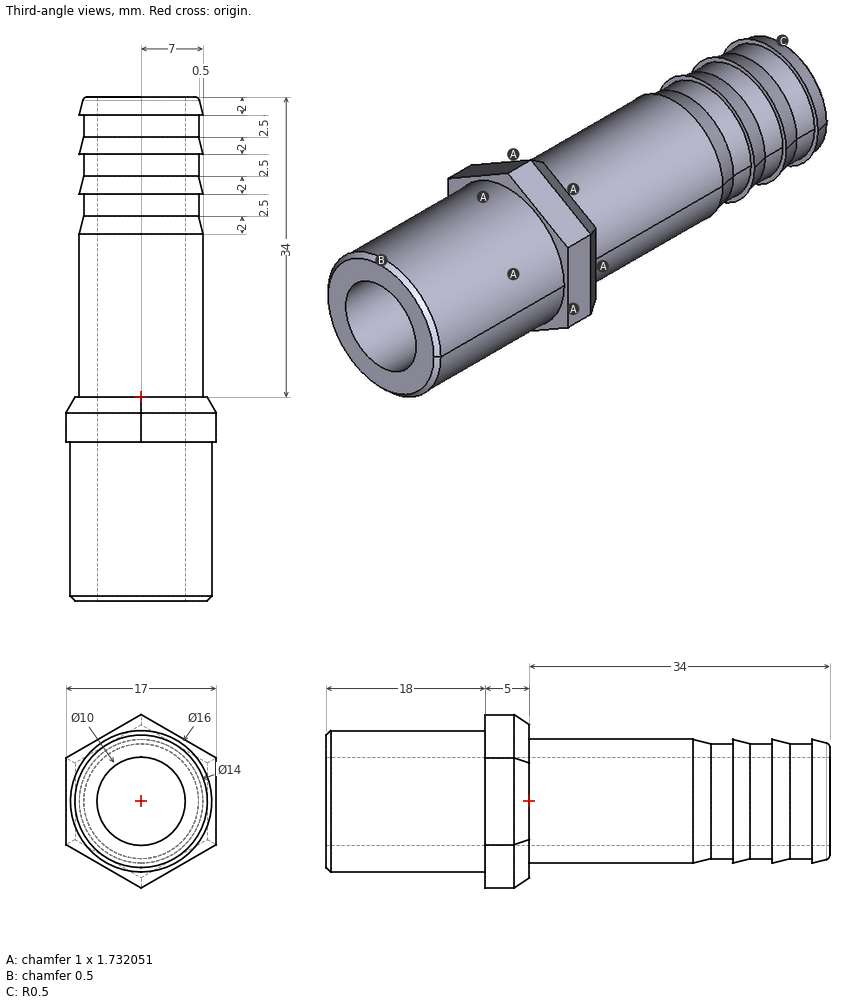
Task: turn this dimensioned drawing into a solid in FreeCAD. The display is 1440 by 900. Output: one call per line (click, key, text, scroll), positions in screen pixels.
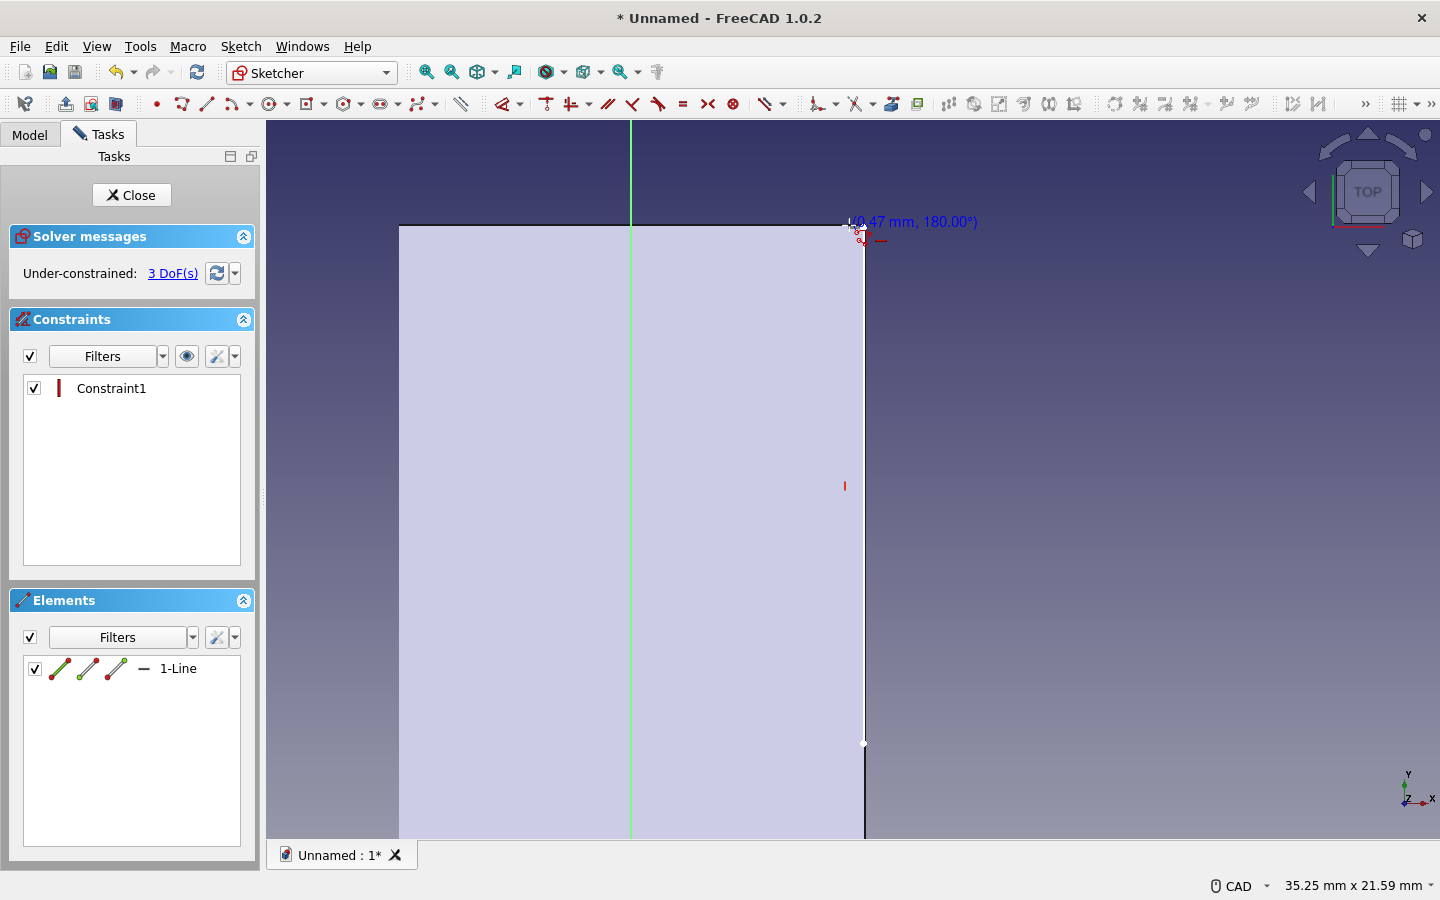
click(848, 225)
click(865, 292)
click(848, 292)
click(848, 375)
click(865, 441)
click(848, 441)
click(848, 525)
click(865, 591)
click(848, 591)
click(848, 675)
click(864, 743)
key(Escape)
key(Escape)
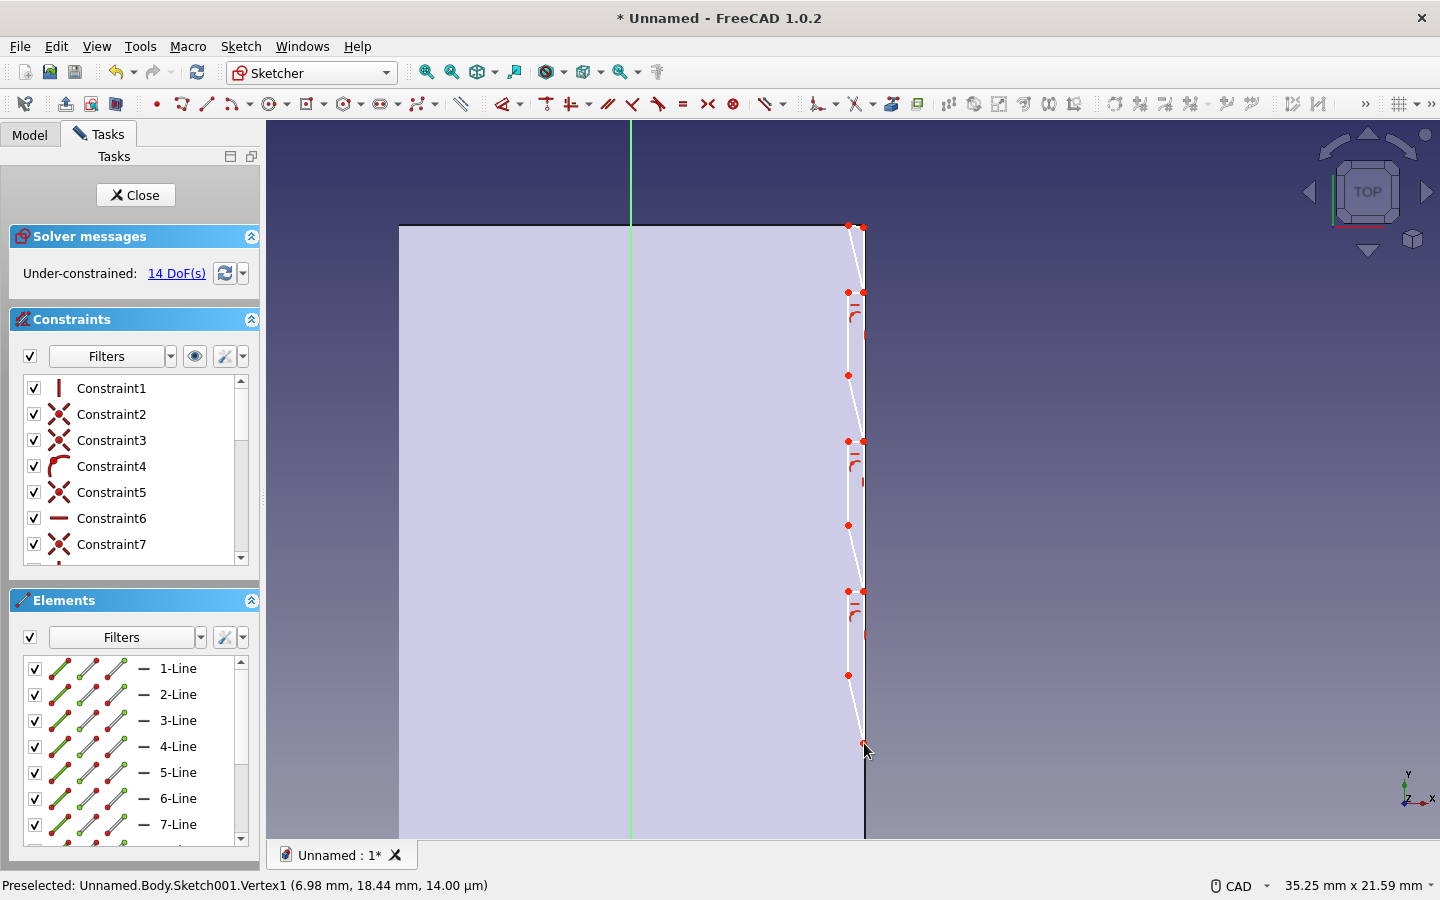
scroll(856, 227, up, 3)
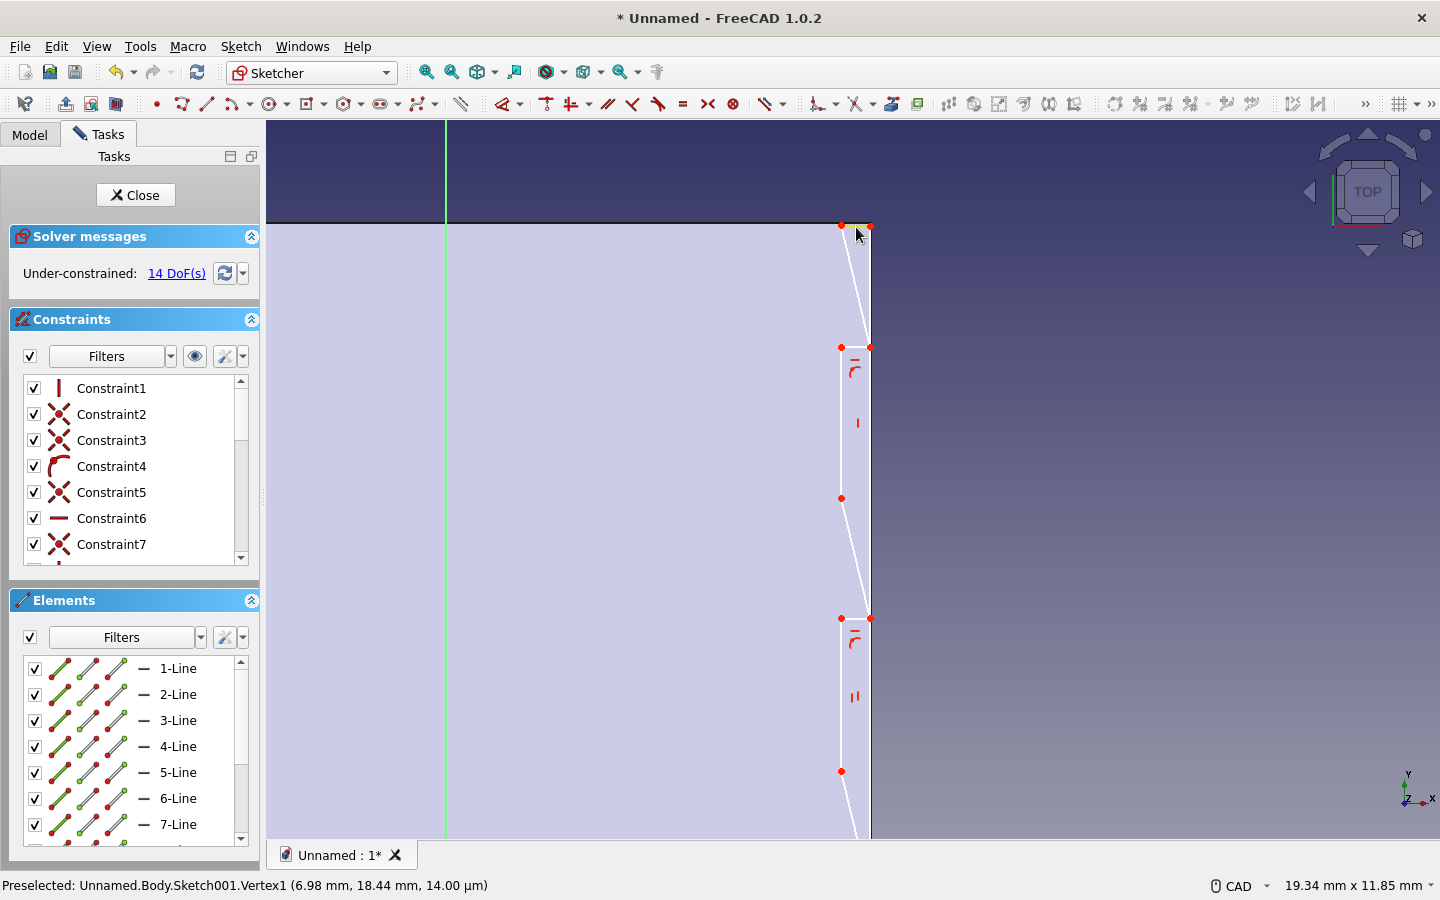
click(856, 226)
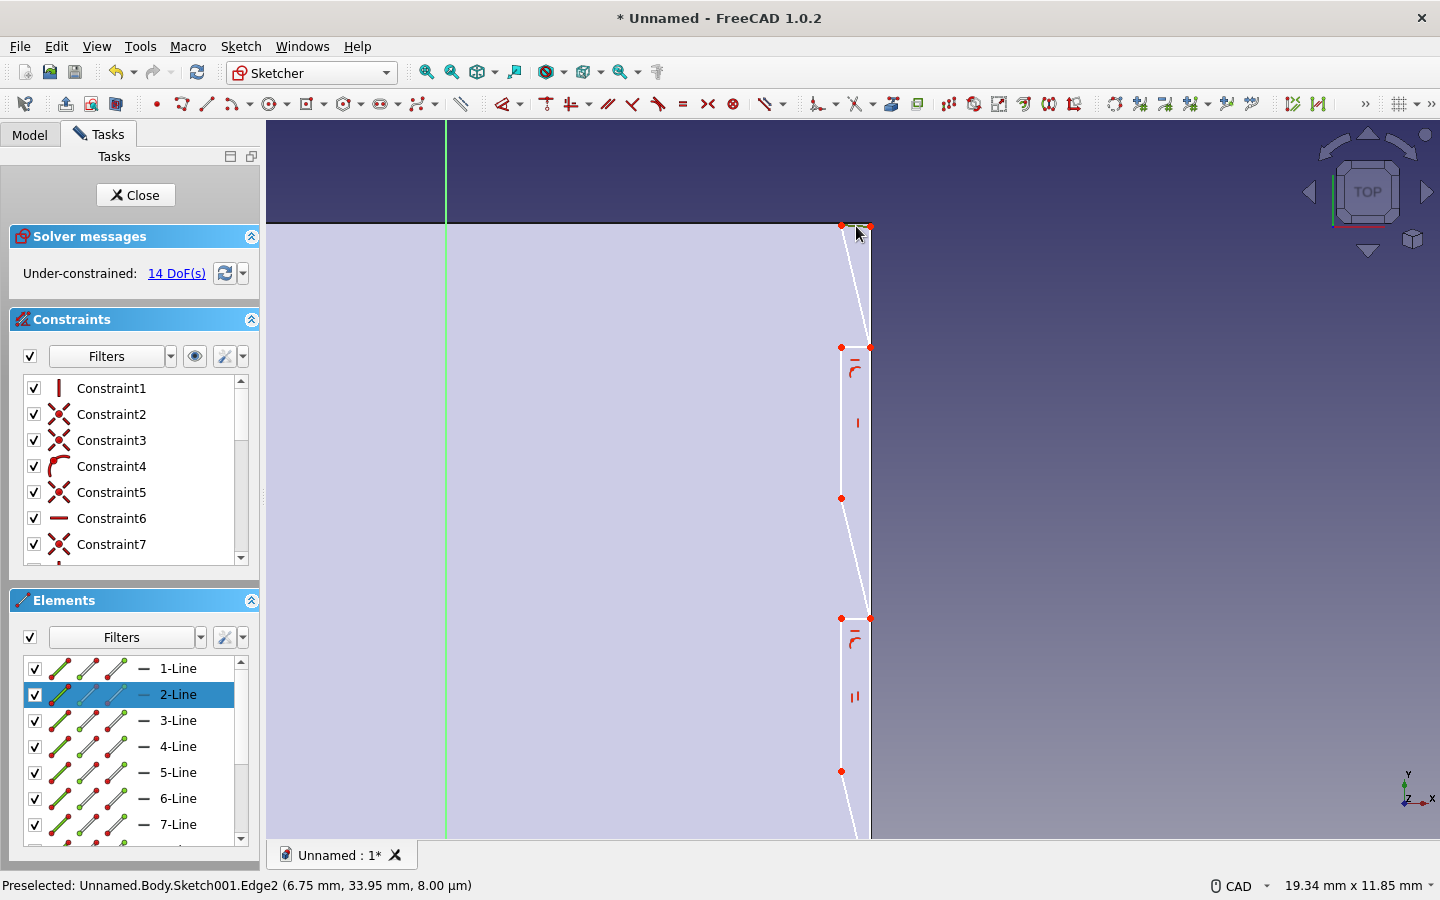
click(588, 104)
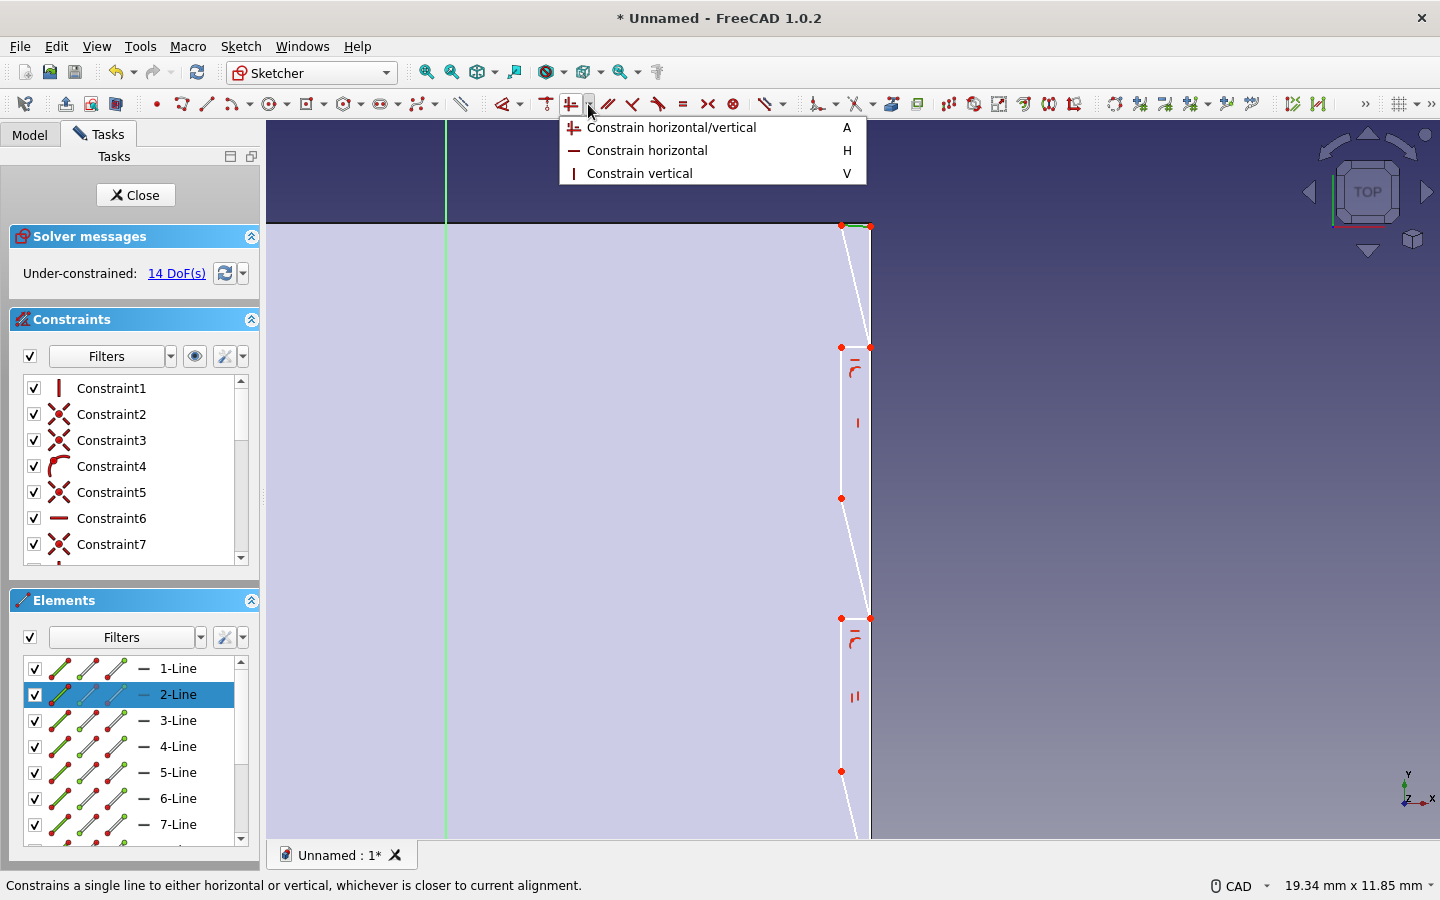
click(713, 150)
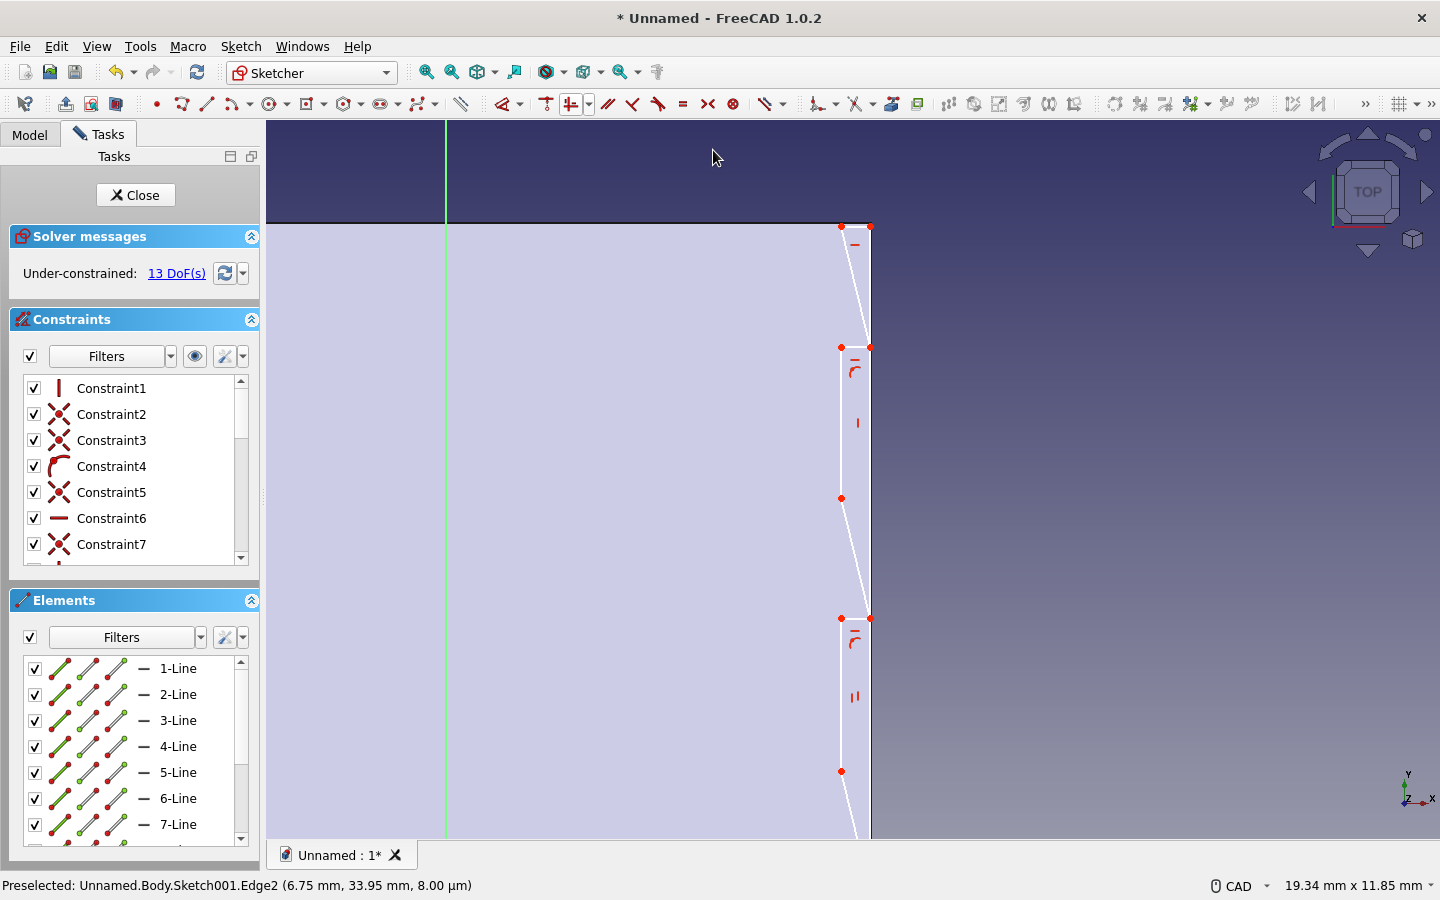
click(502, 104)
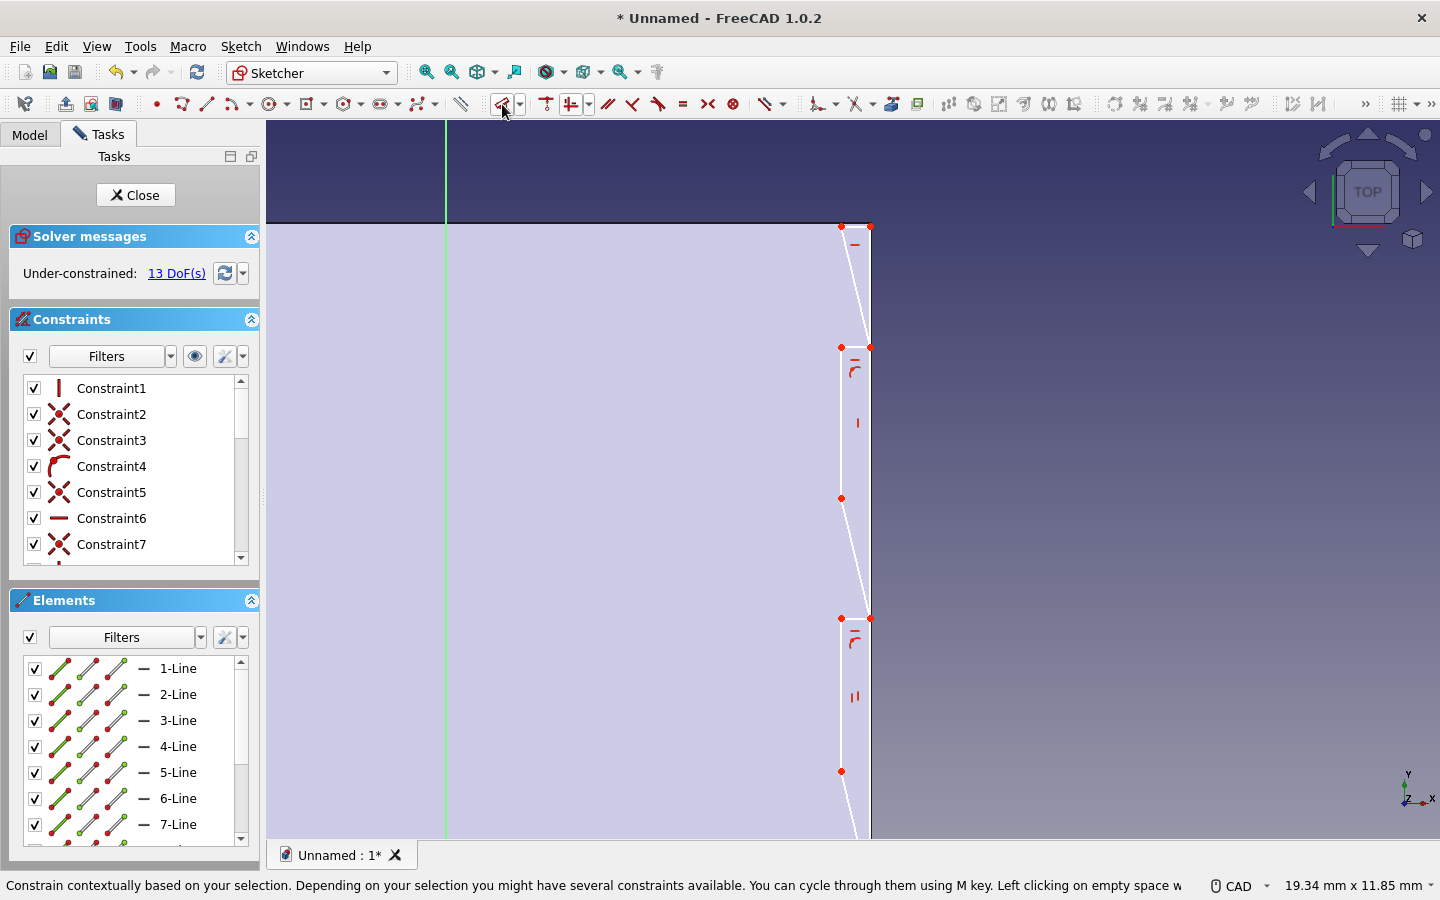
scroll(826, 226, down, 7)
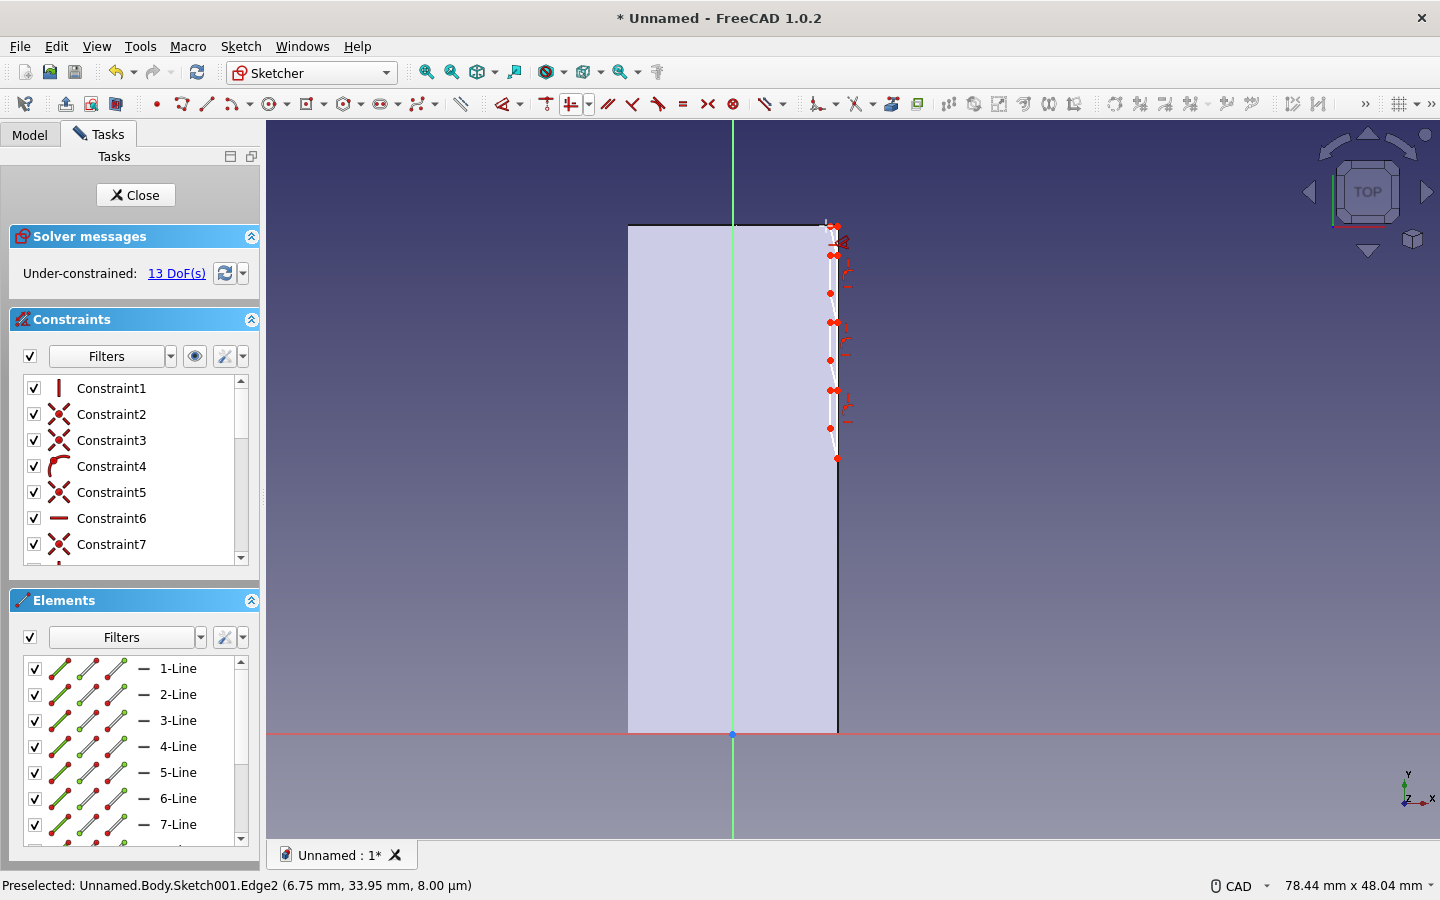
click(837, 458)
click(785, 768)